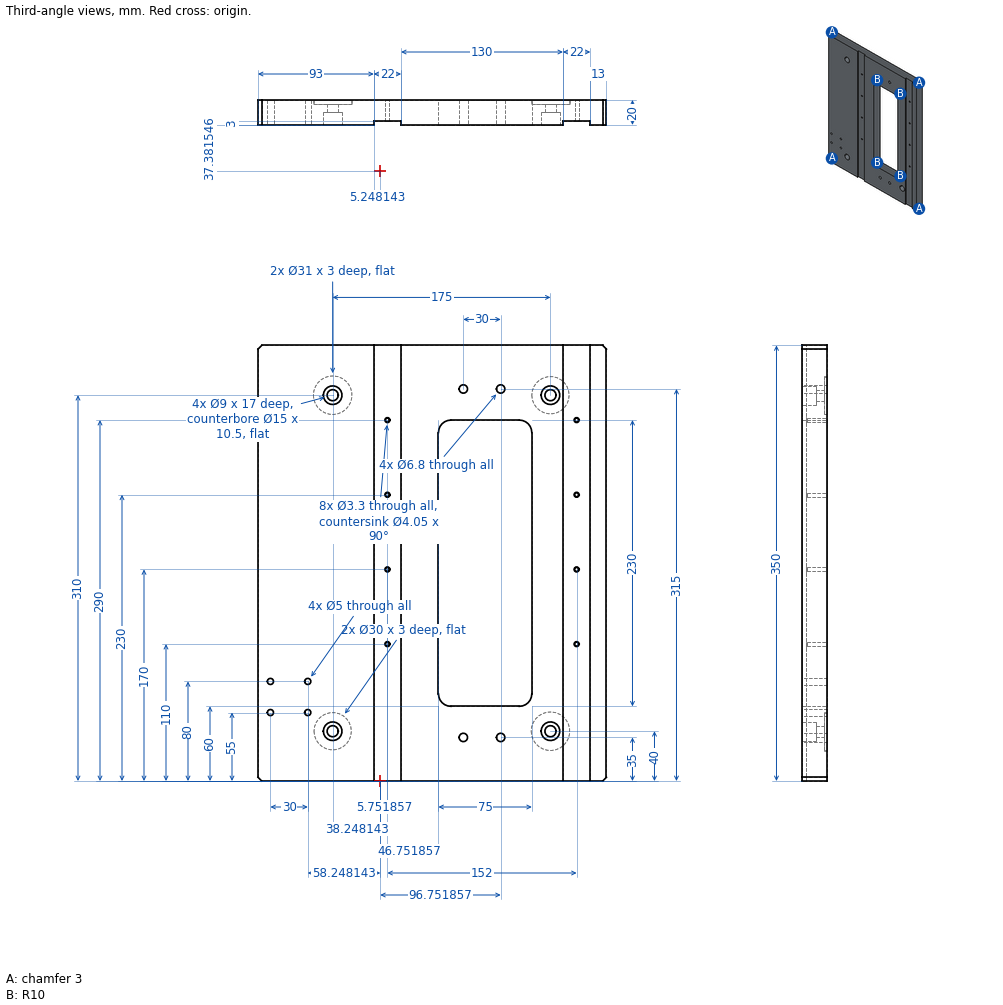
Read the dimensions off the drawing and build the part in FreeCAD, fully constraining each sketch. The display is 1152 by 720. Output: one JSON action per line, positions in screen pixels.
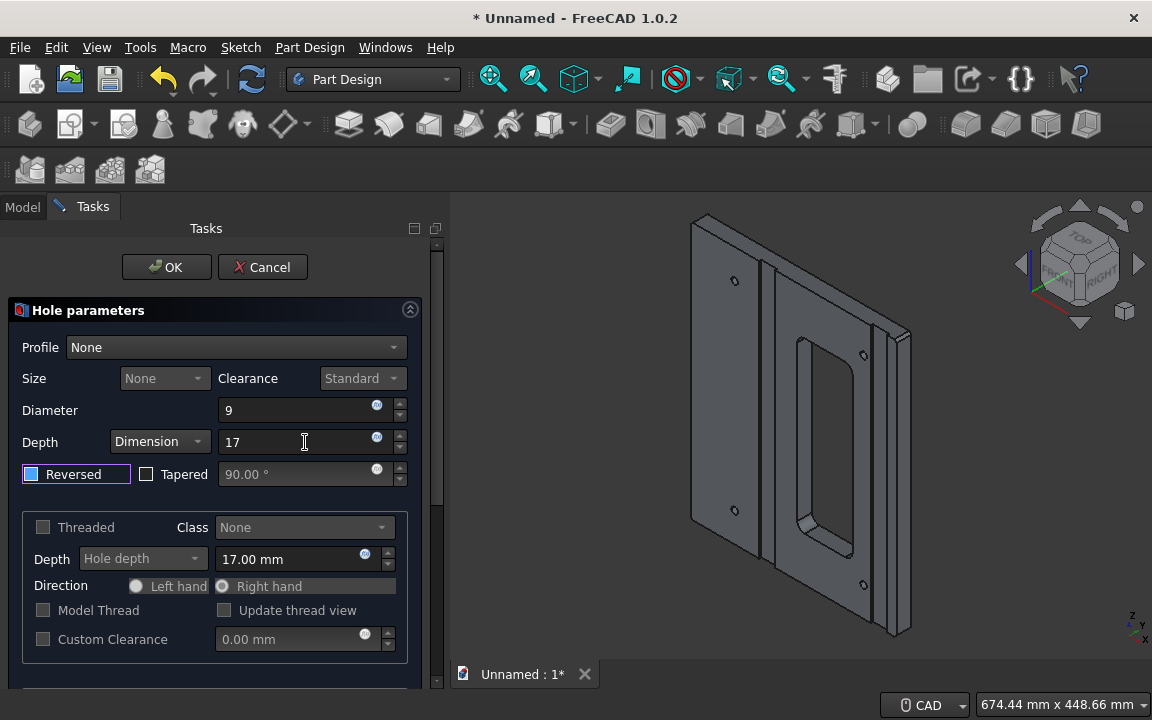
{"action": "scroll", "coordinate": [437, 463], "scroll_direction": "down", "scroll_amount": 2}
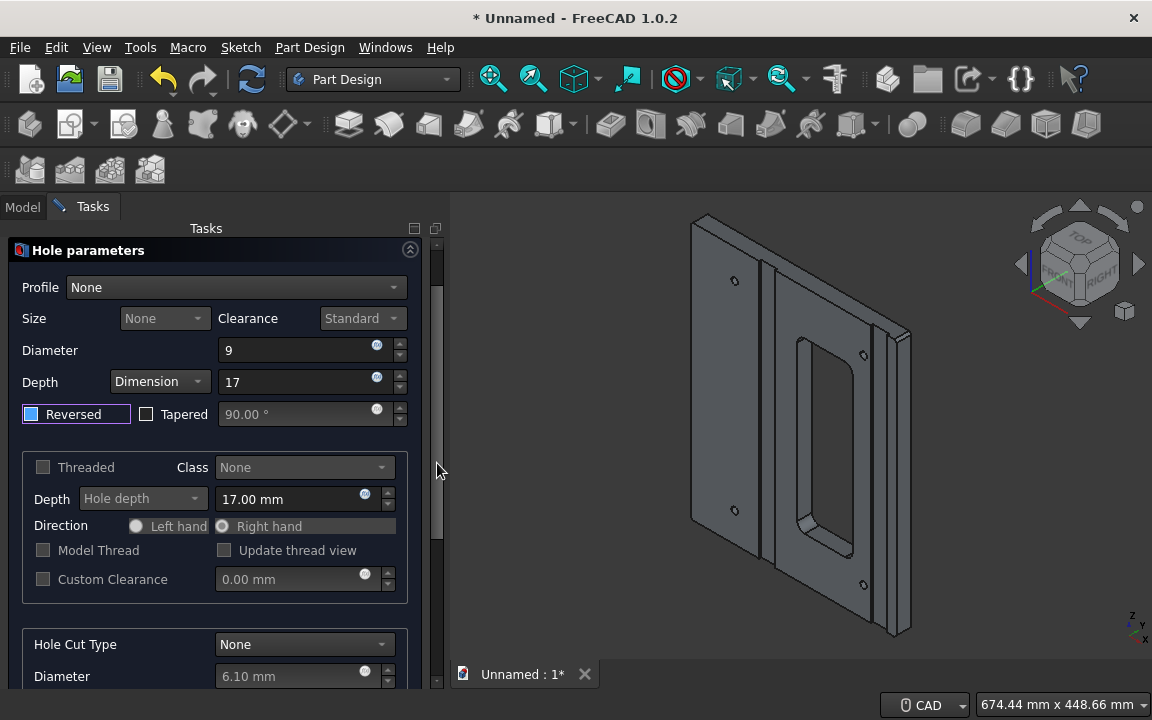
{"action": "left_click", "coordinate": [306, 584]}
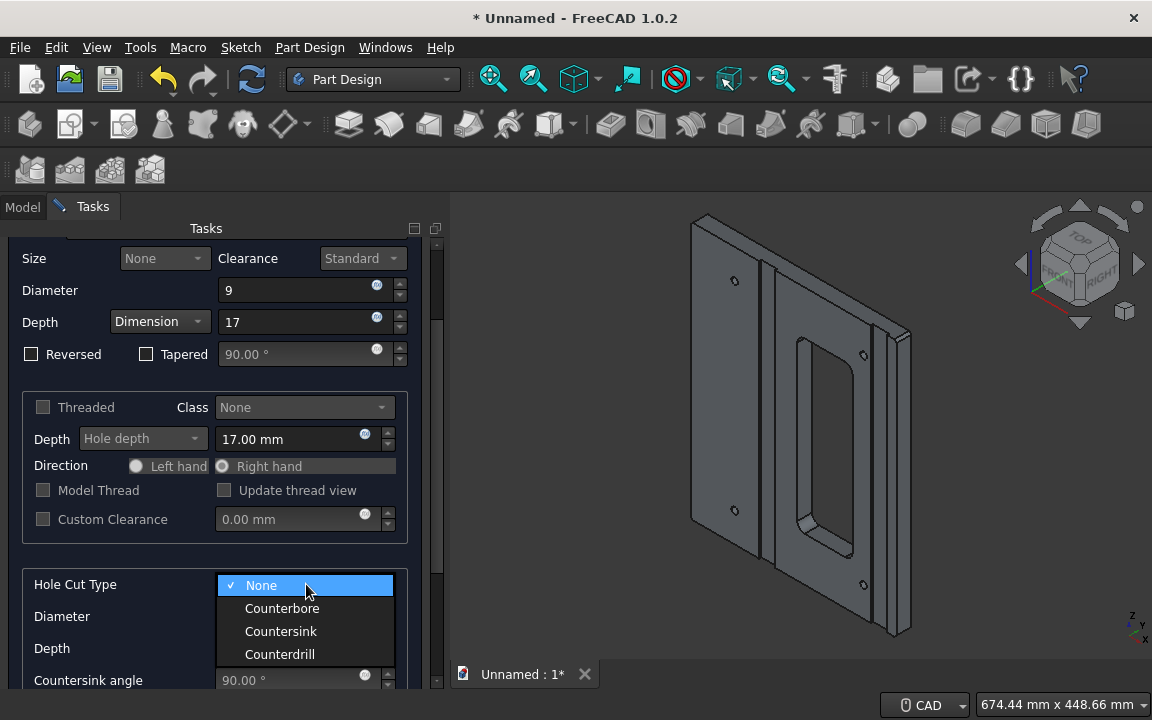
{"action": "left_click", "coordinate": [304, 608]}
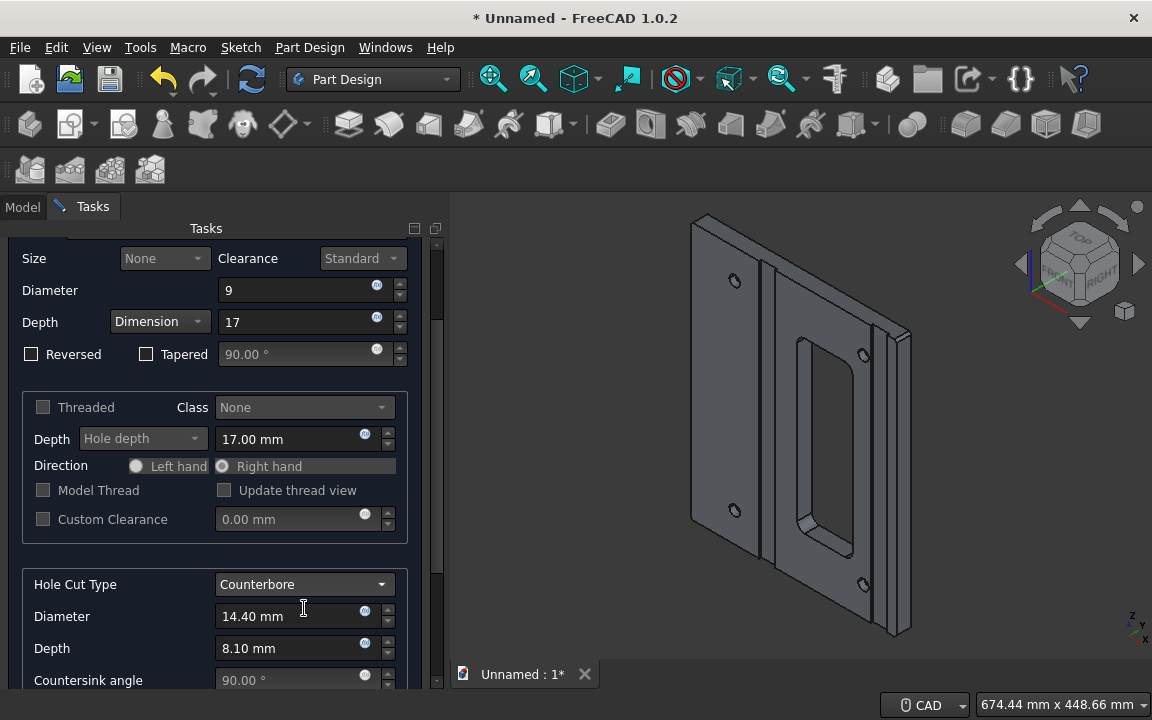
{"action": "triple_click", "coordinate": [298, 616]}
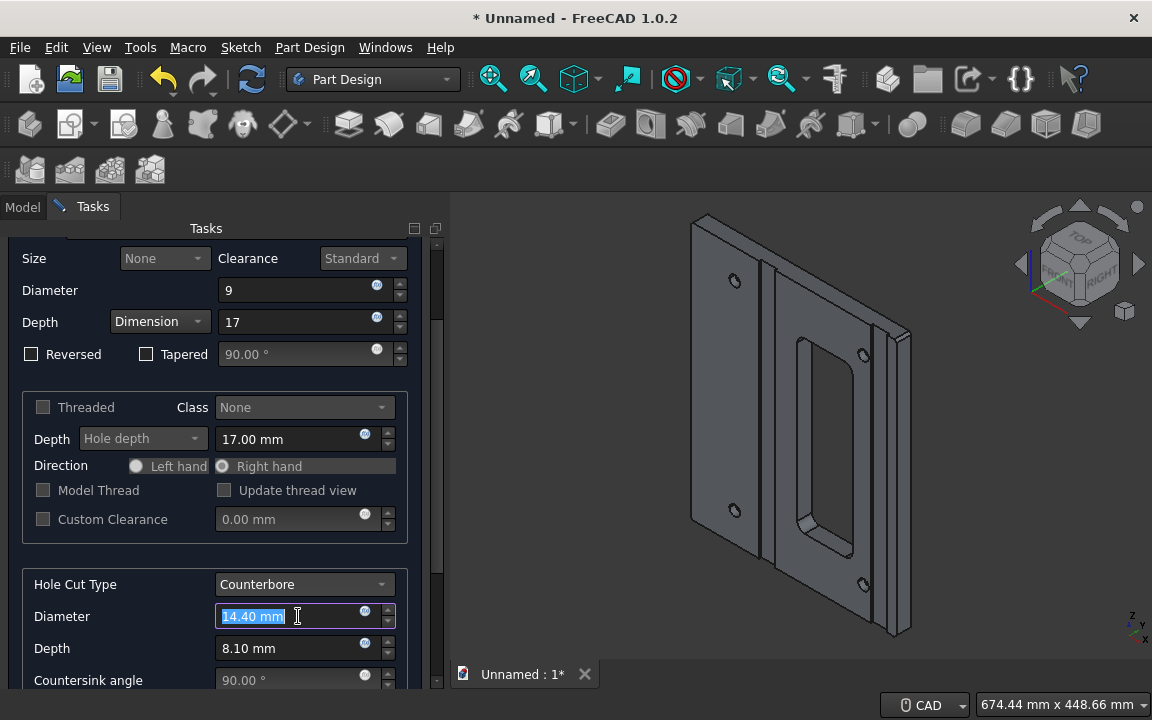
{"action": "type", "text": "15"}
{"action": "key", "text": "Tab"}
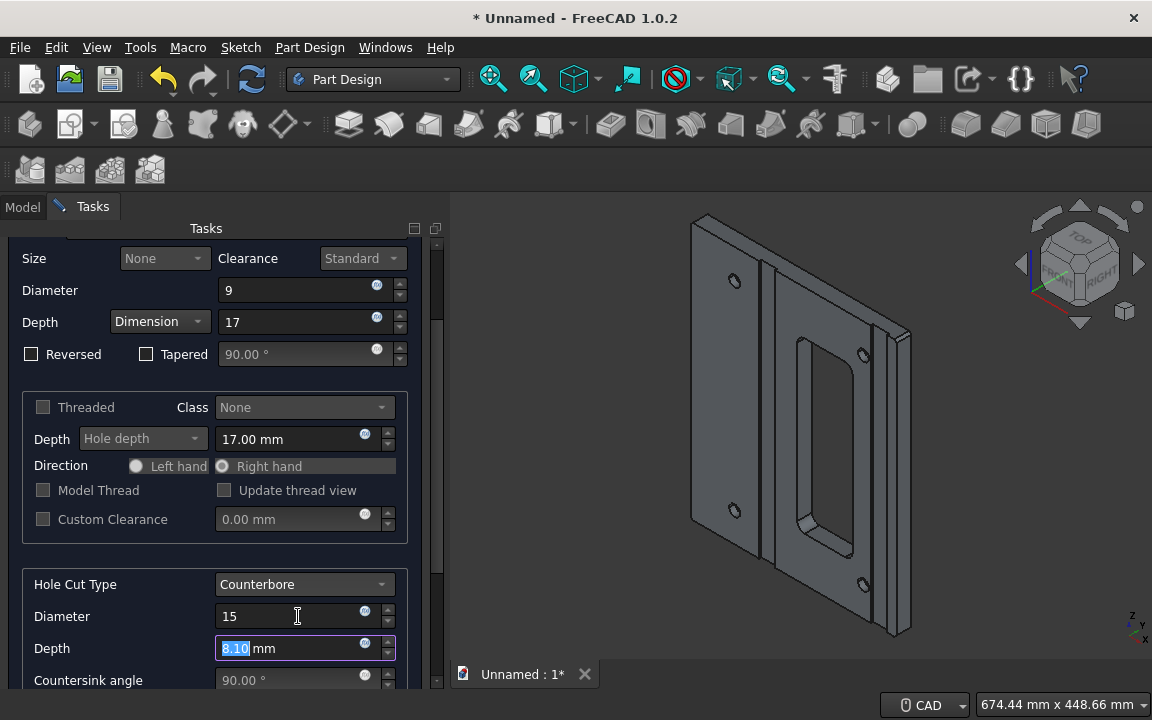
{"action": "type", "text": "10.5"}
{"action": "key", "text": "Tab"}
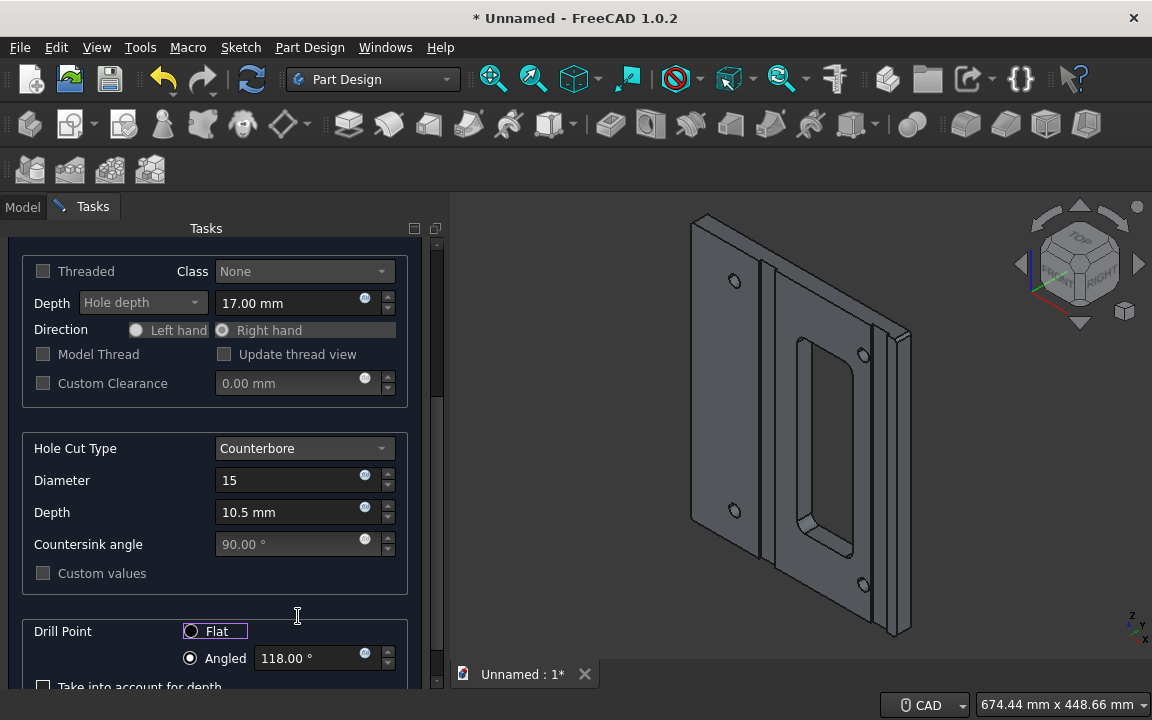
{"action": "left_click", "coordinate": [191, 631]}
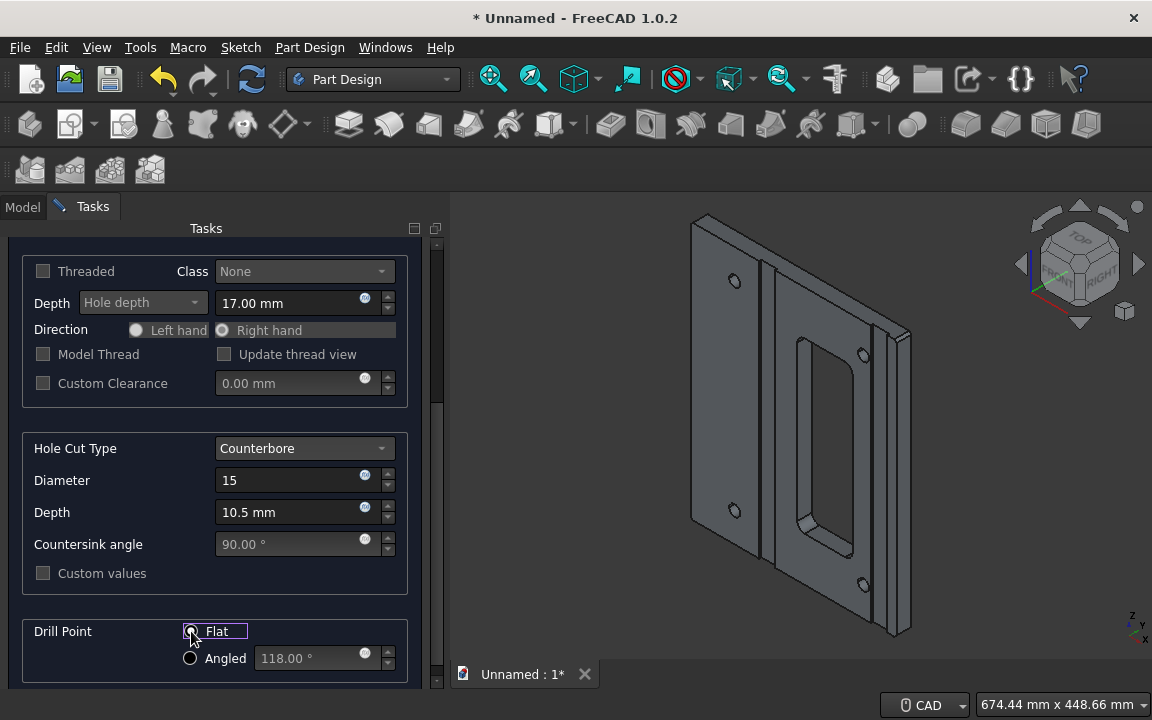
{"action": "scroll", "coordinate": [437, 463], "scroll_direction": "up", "scroll_amount": 6}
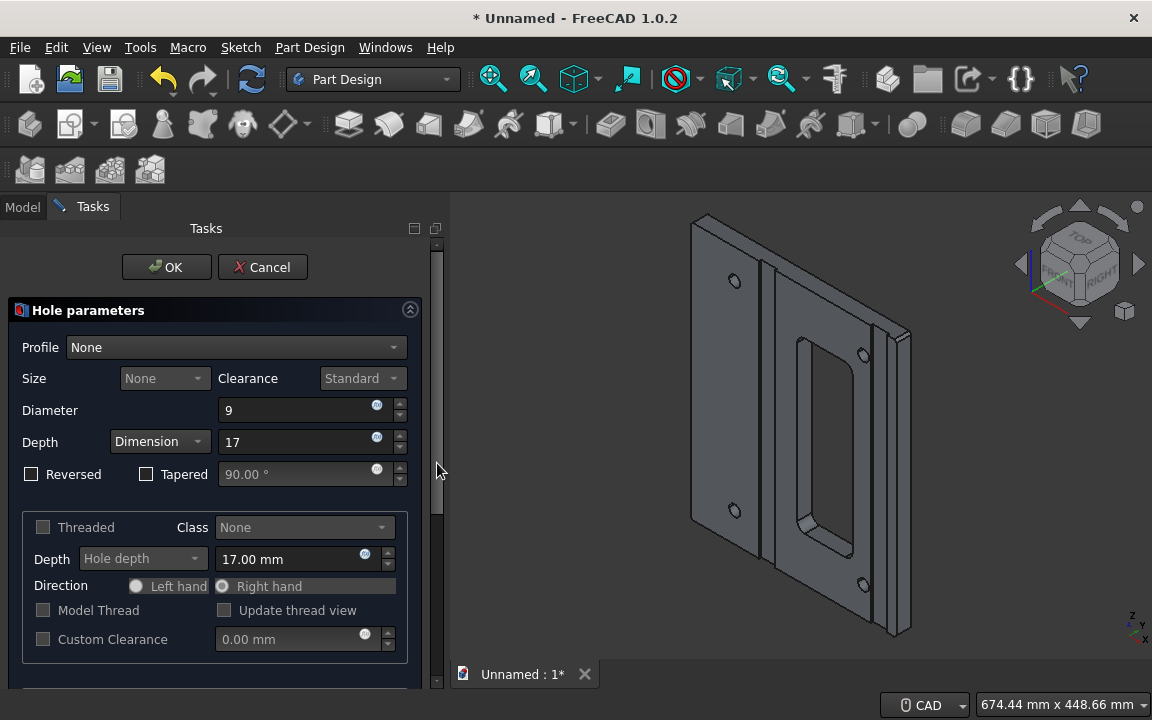
{"action": "left_click", "coordinate": [167, 267]}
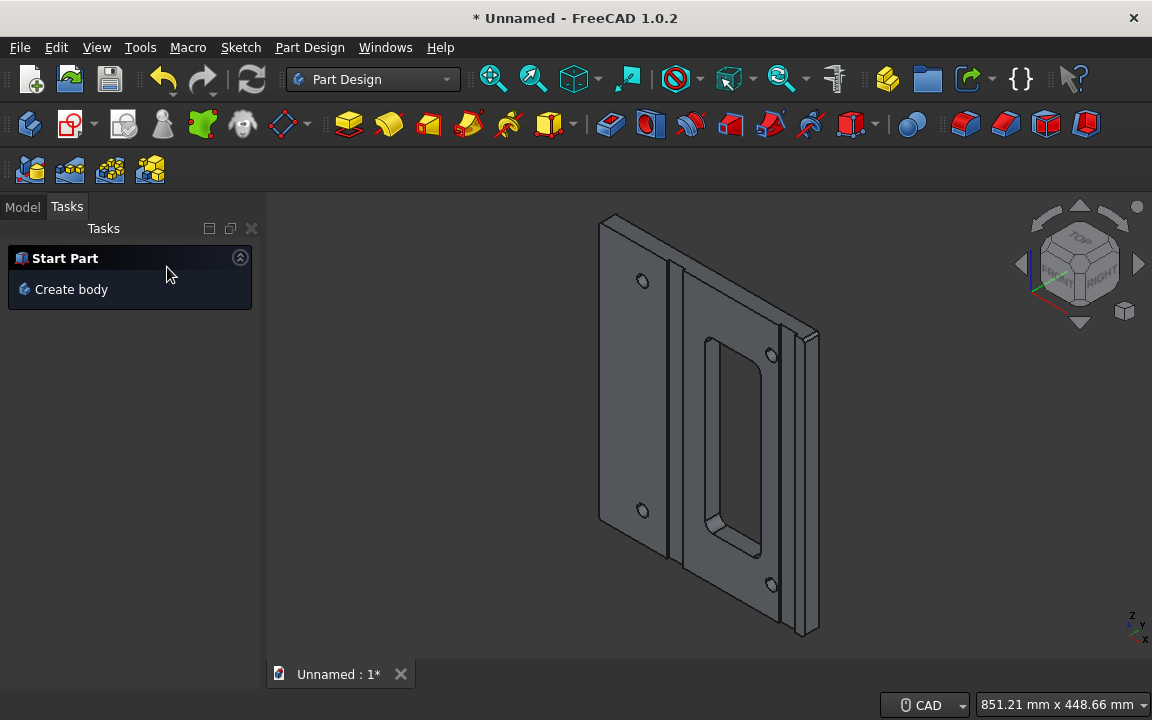
{"action": "key", "text": "1"}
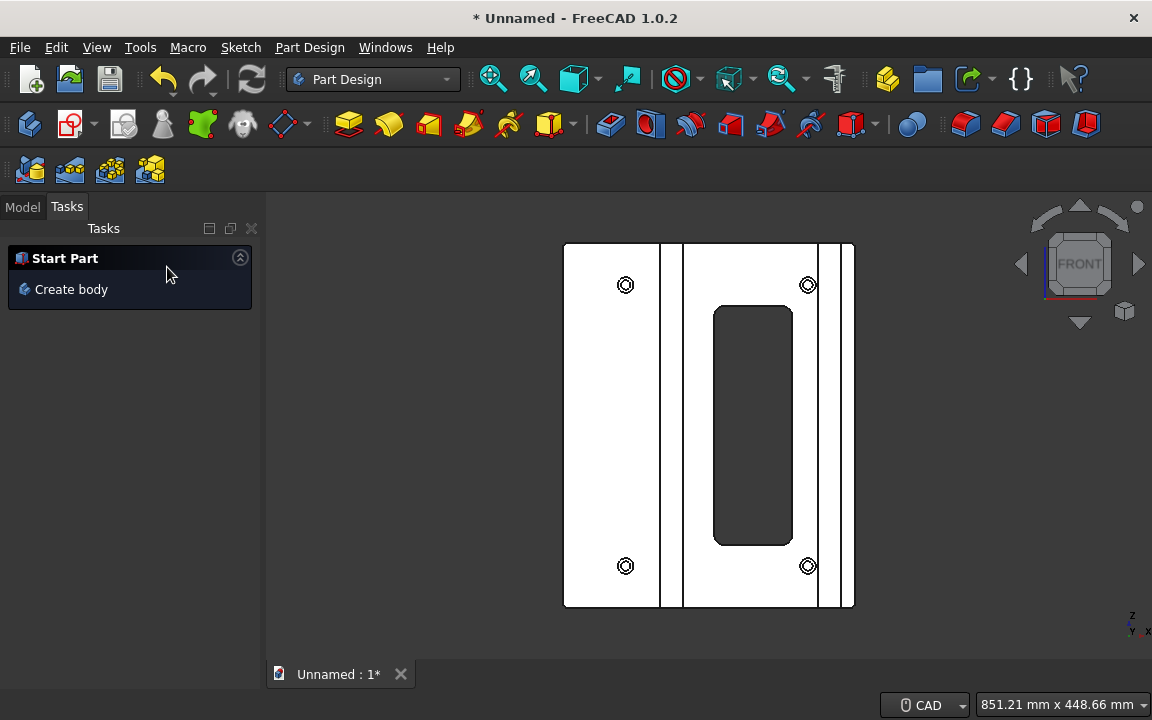
{"action": "left_click", "coordinate": [672, 268]}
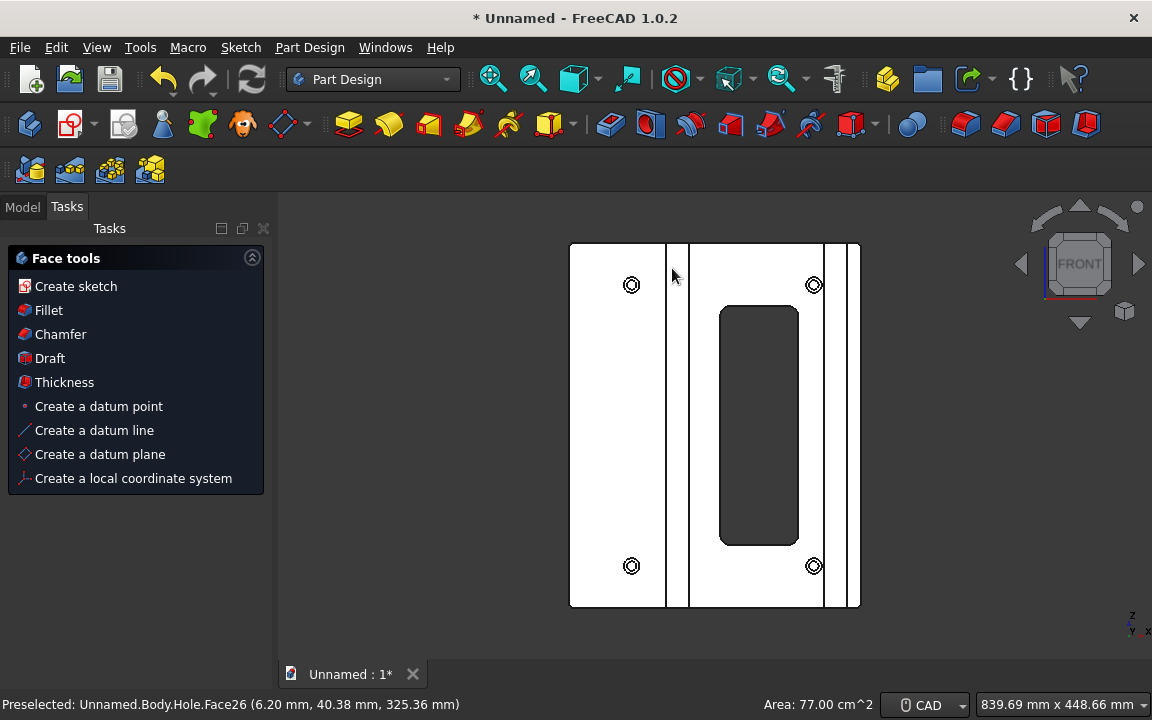
{"action": "left_click", "coordinate": [70, 124]}